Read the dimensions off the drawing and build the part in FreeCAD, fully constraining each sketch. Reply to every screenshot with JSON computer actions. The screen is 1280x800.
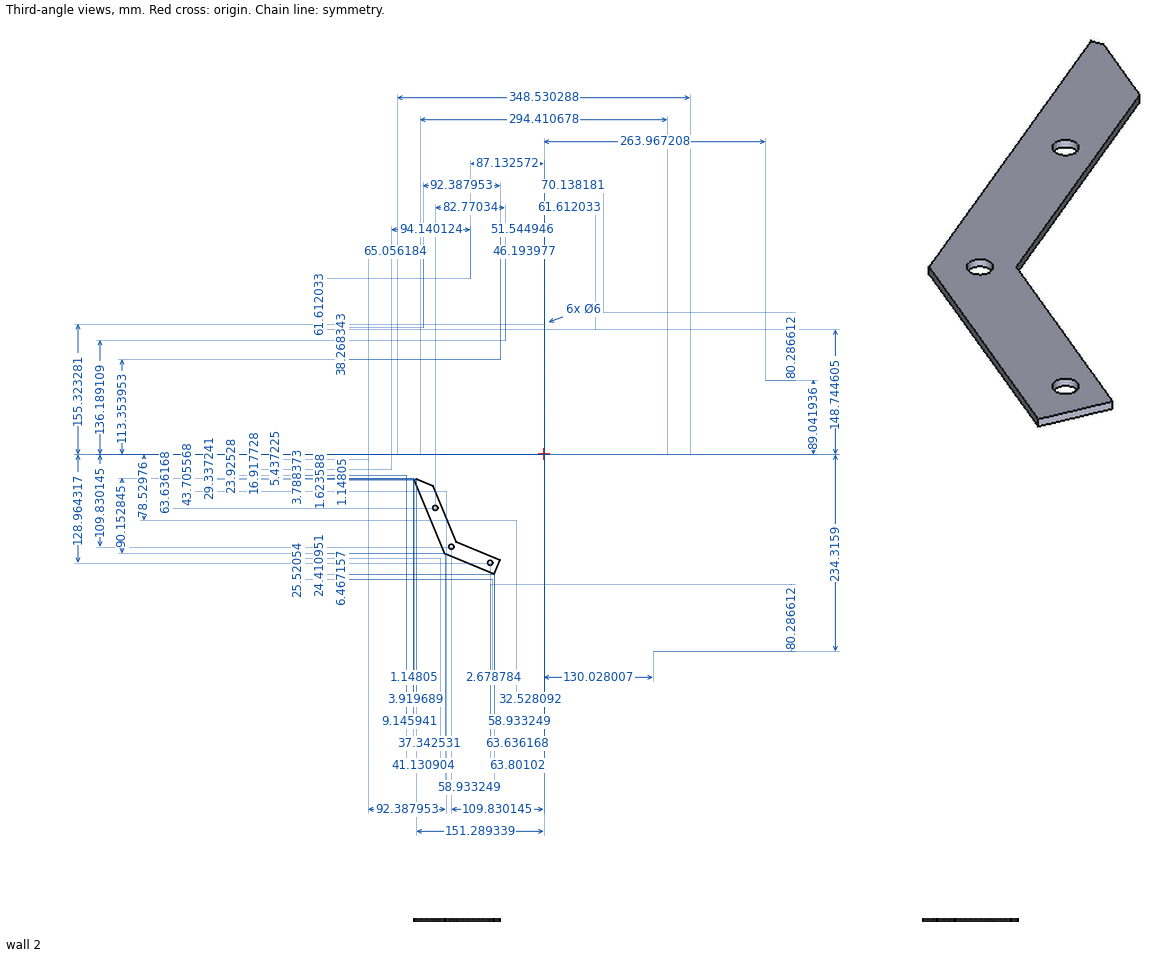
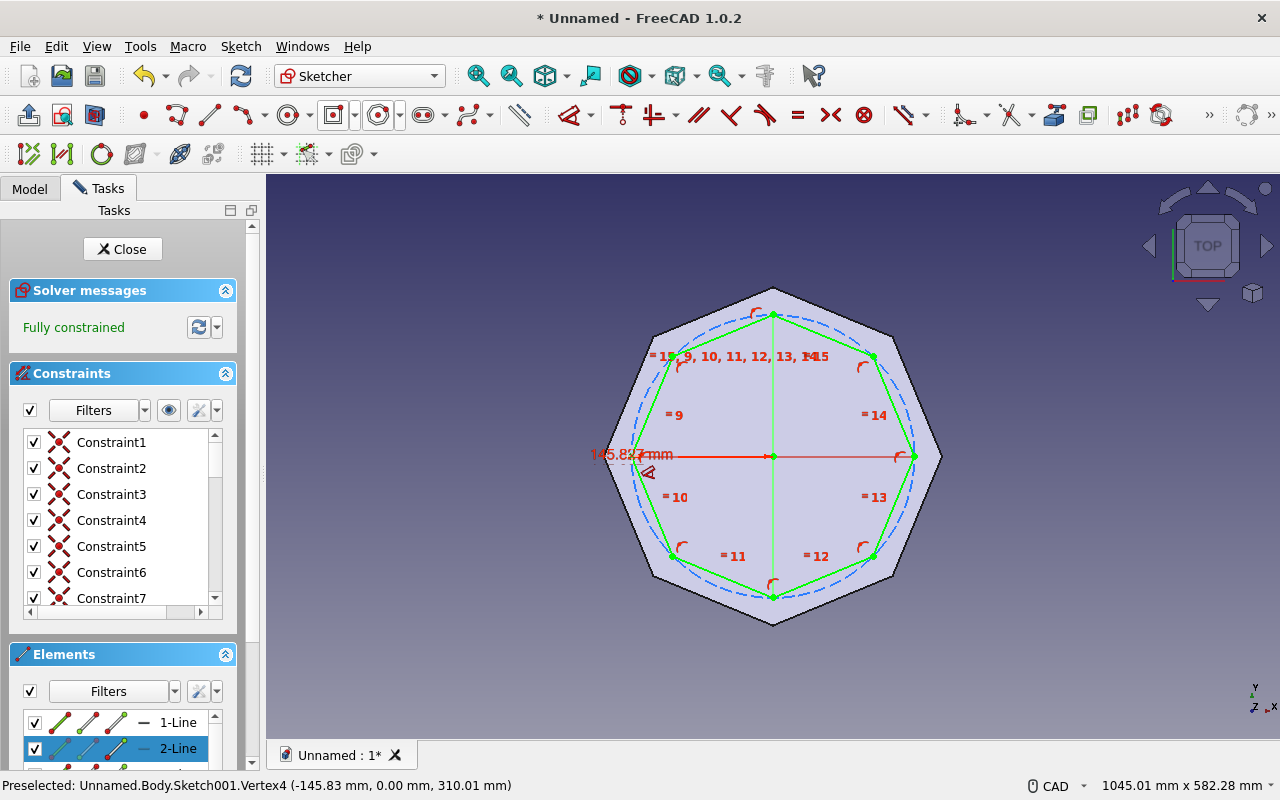
{"action": "left_click", "coordinate": [914, 456]}
{"action": "left_click", "coordinate": [708, 490]}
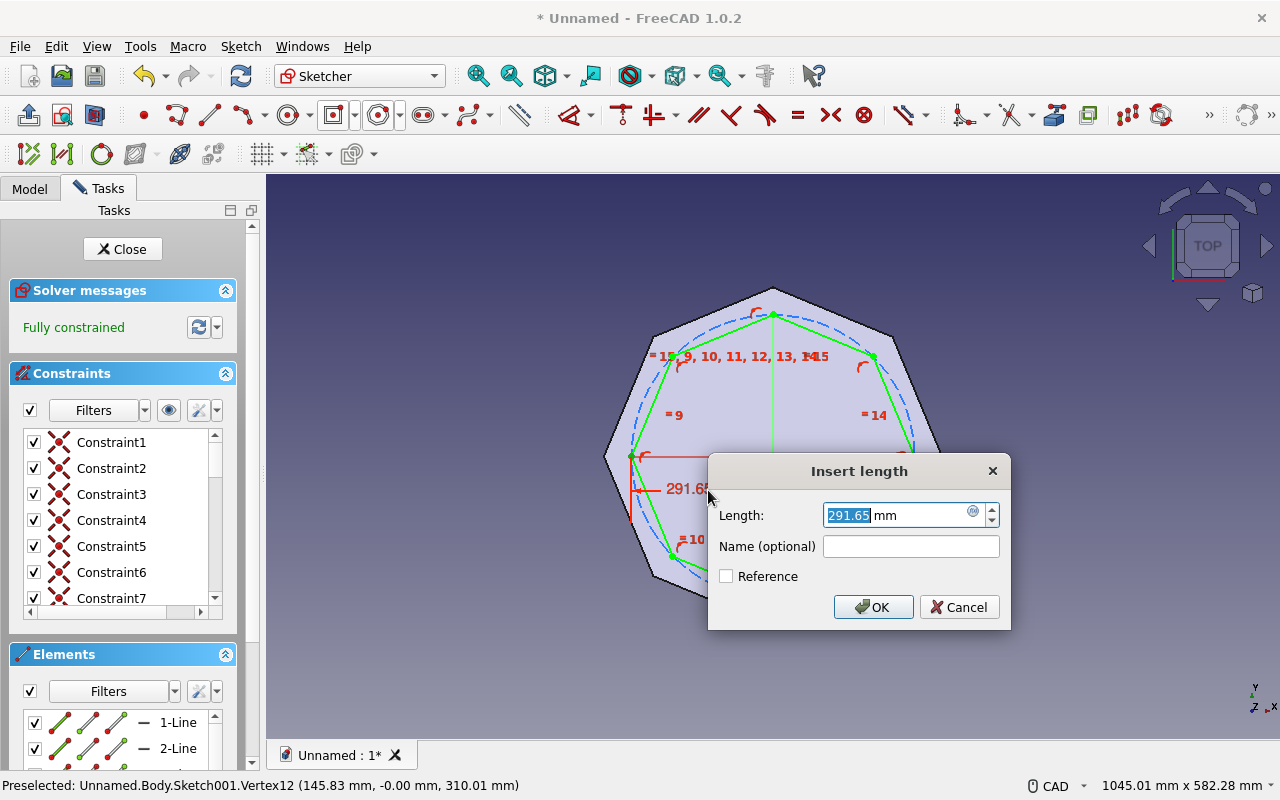
{"action": "type", "text": "294.410678"}
{"action": "key", "text": "Return"}
{"action": "key", "text": "Escape"}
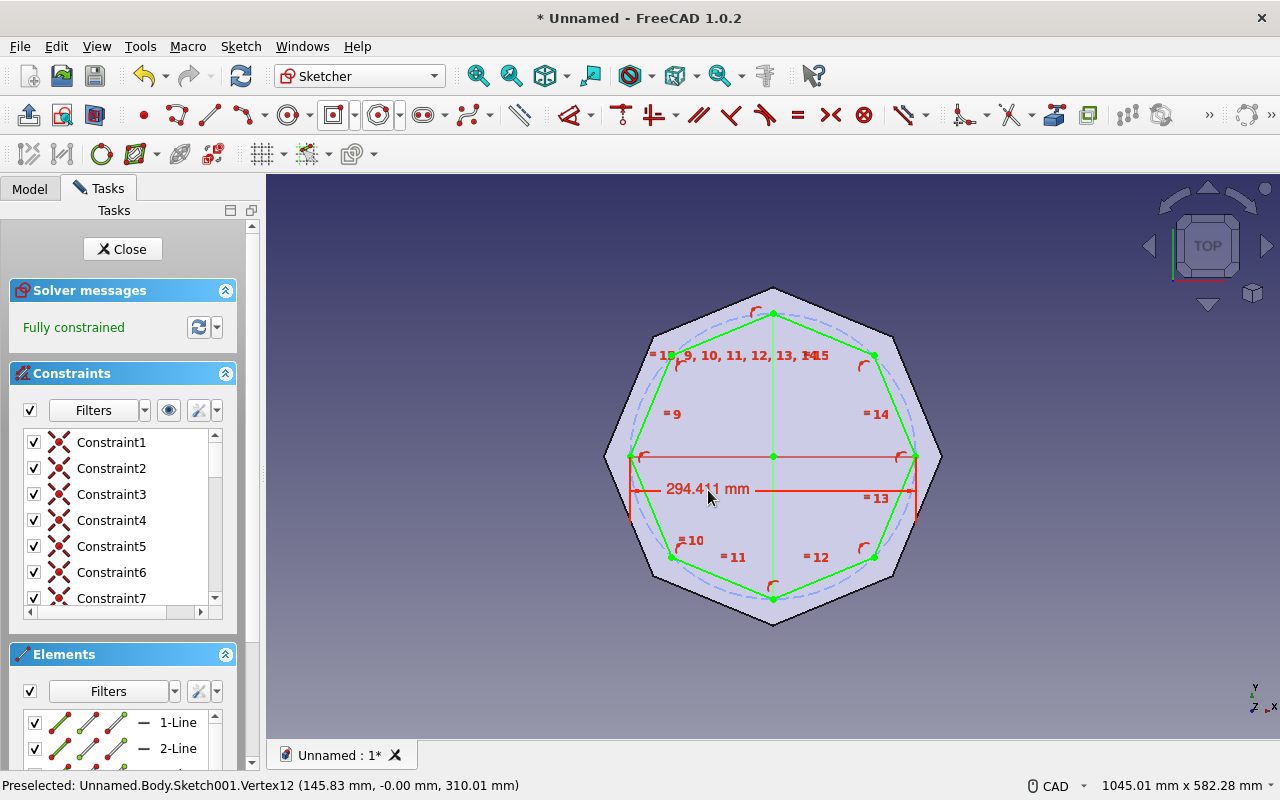
{"action": "left_click", "coordinate": [123, 249]}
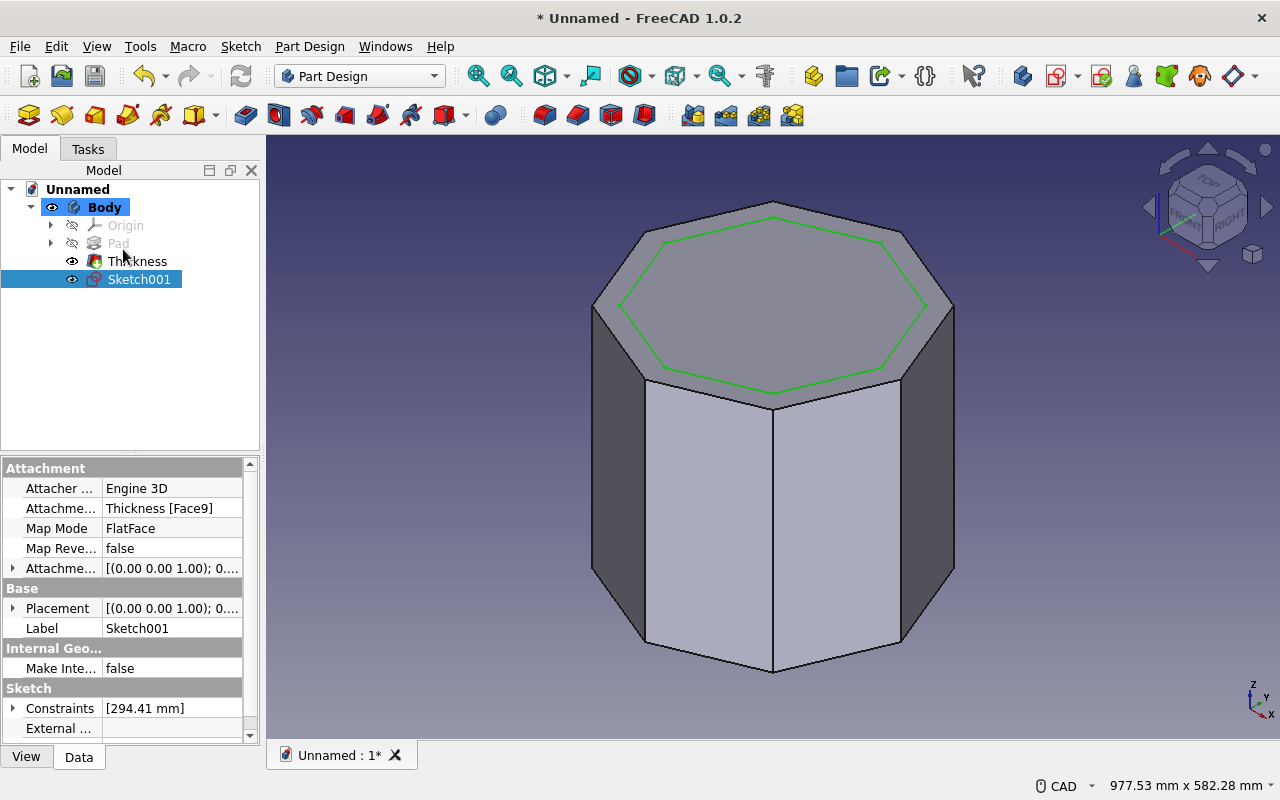
{"action": "left_click", "coordinate": [246, 116]}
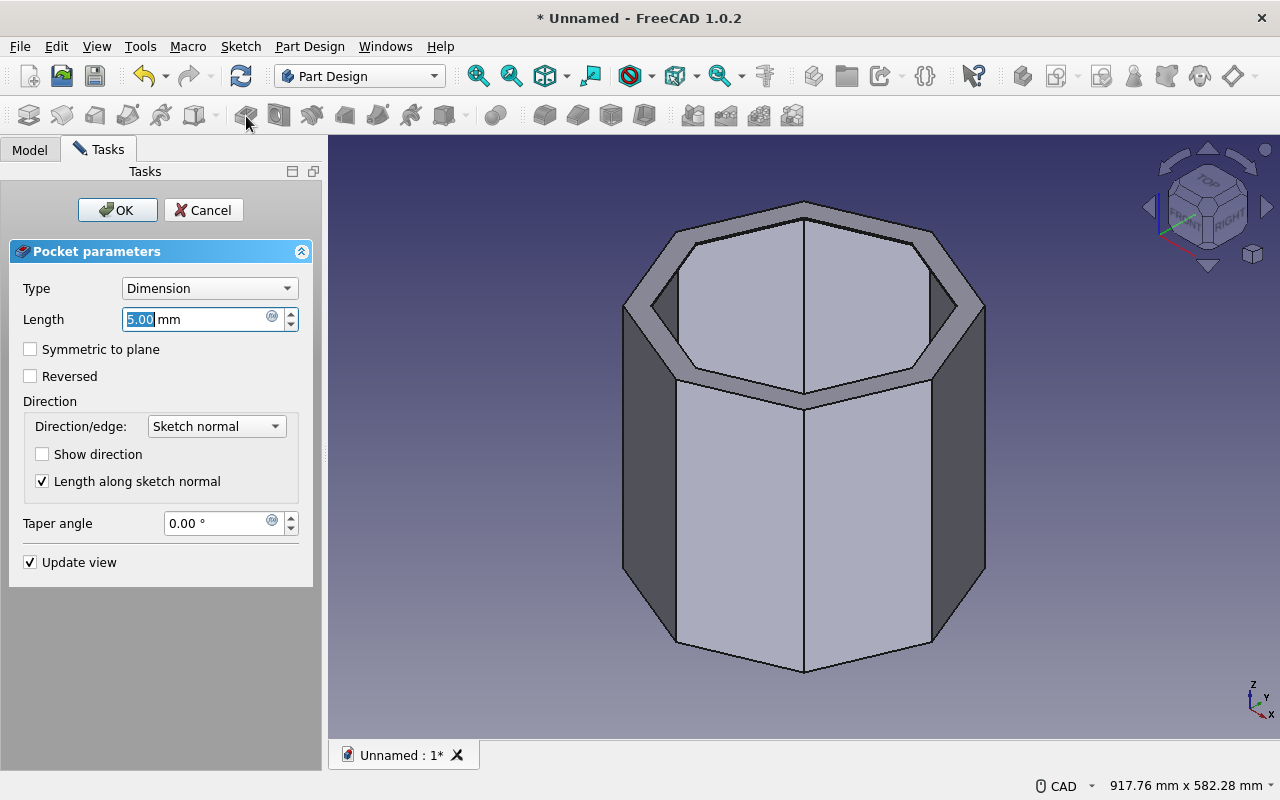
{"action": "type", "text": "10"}
{"action": "key", "text": "Tab"}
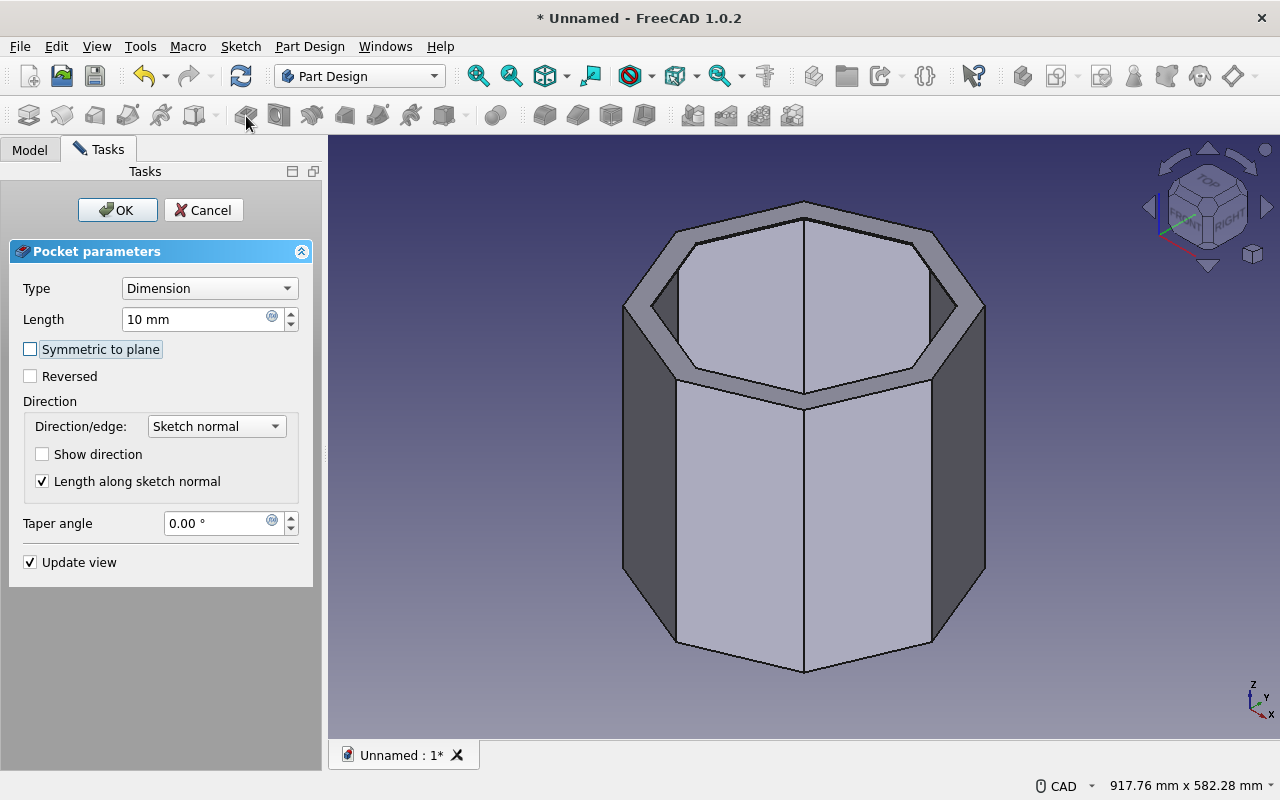
{"action": "left_click", "coordinate": [118, 210]}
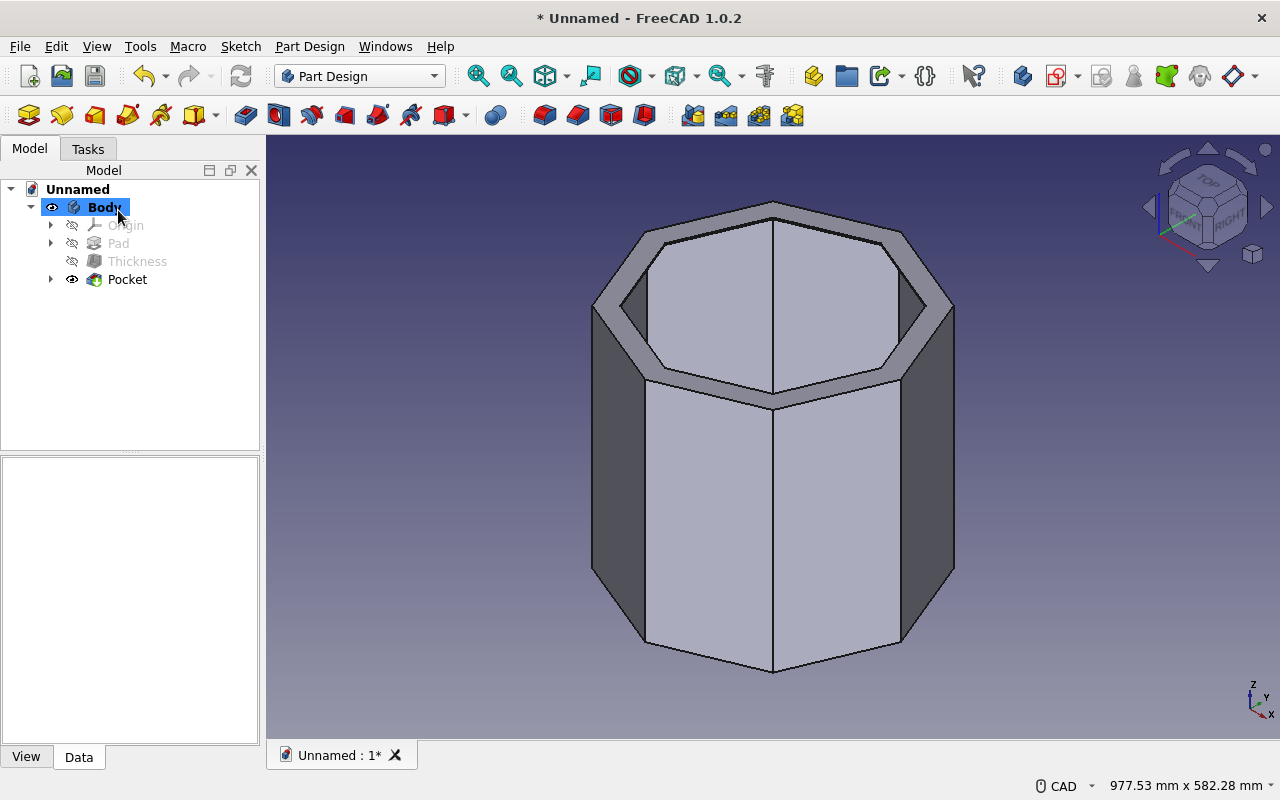
{"action": "scroll", "coordinate": [627, 263], "scroll_direction": "up", "scroll_amount": 6}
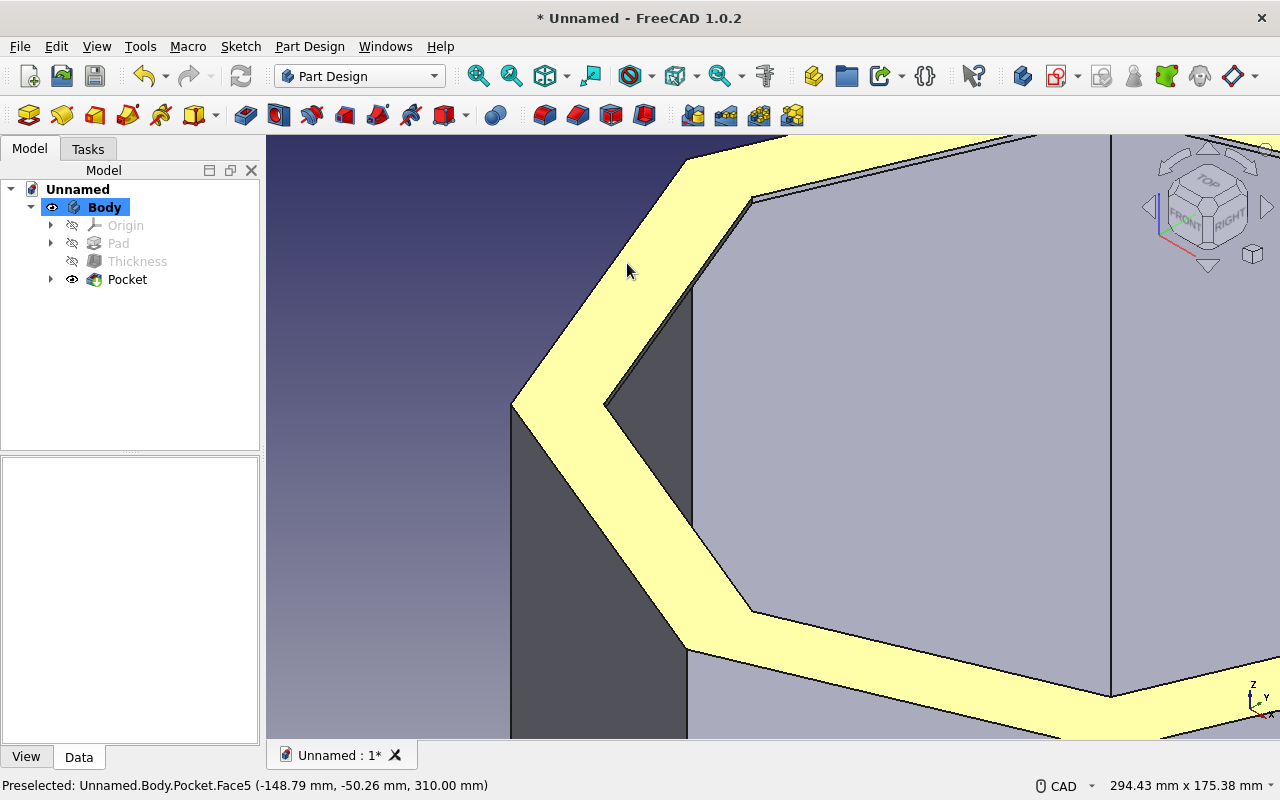
{"action": "left_click", "coordinate": [626, 263]}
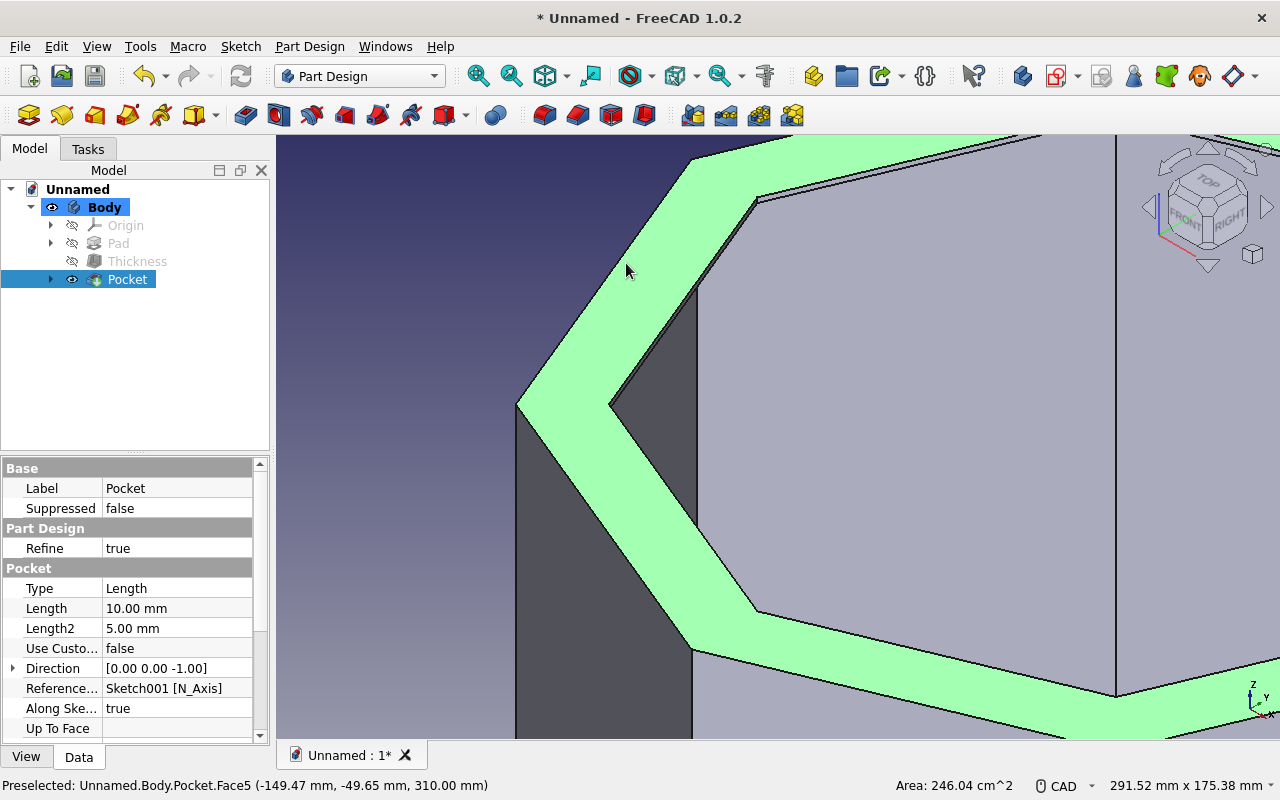
{"action": "left_click", "coordinate": [1056, 76]}